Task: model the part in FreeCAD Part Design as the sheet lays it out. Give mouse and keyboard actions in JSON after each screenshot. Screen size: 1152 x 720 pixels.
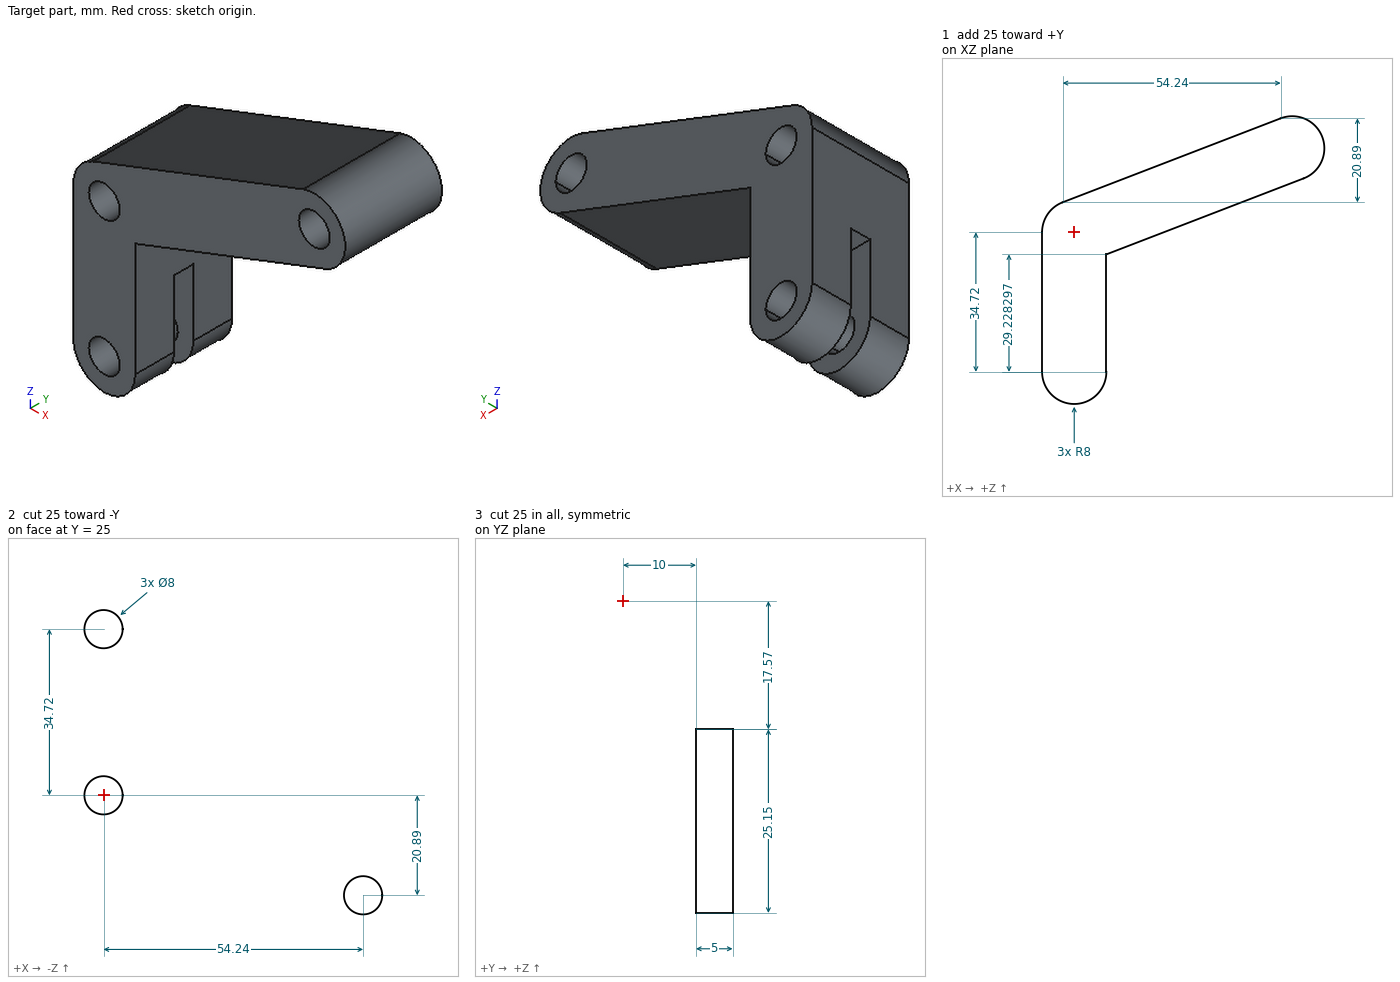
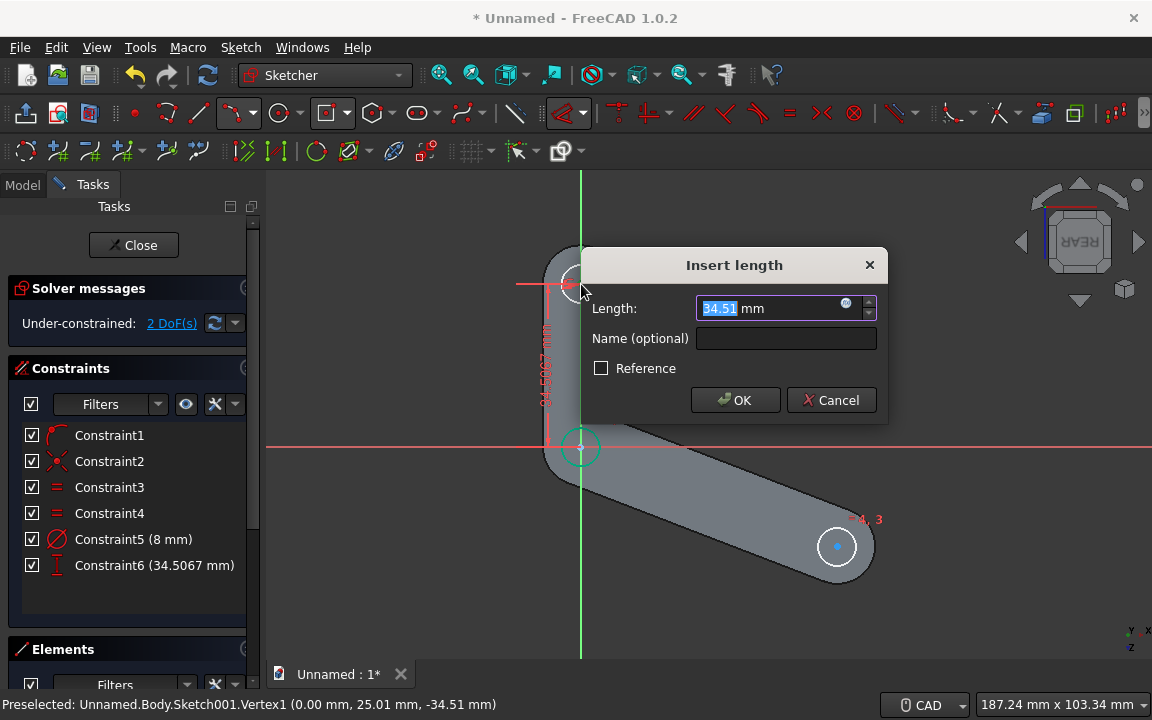
{"action": "type", "text": "34.72"}
{"action": "key", "text": "Return"}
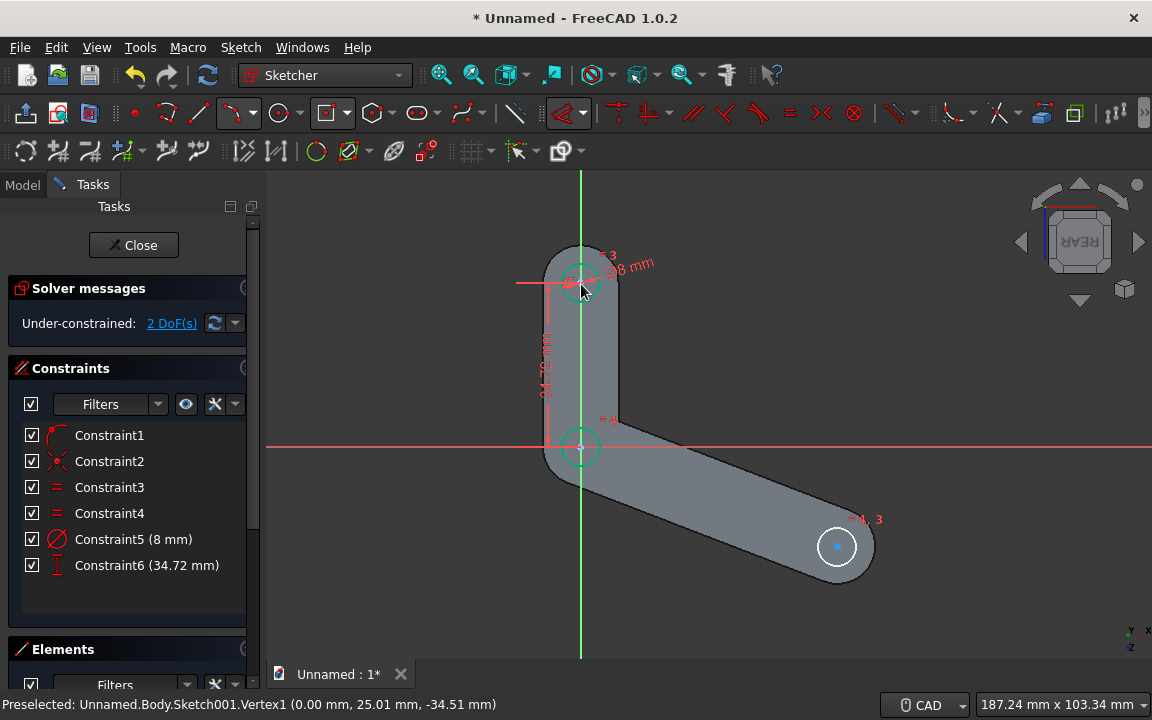
{"action": "left_click", "coordinate": [837, 547]}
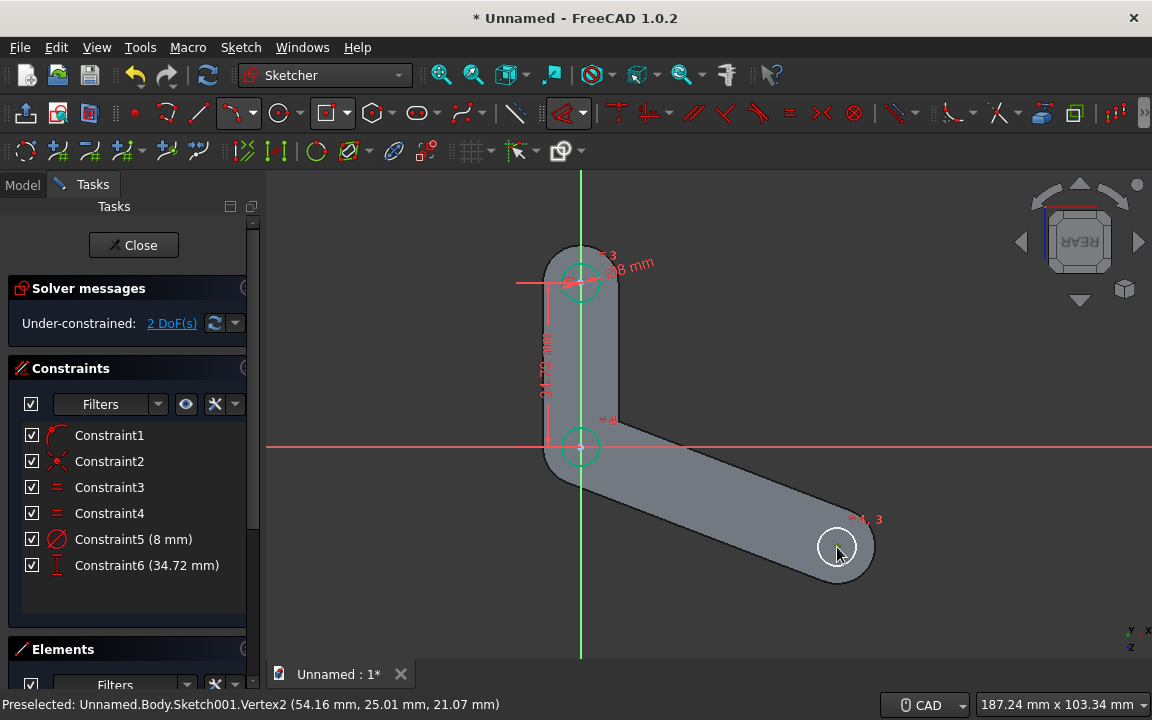
{"action": "key", "text": "l"}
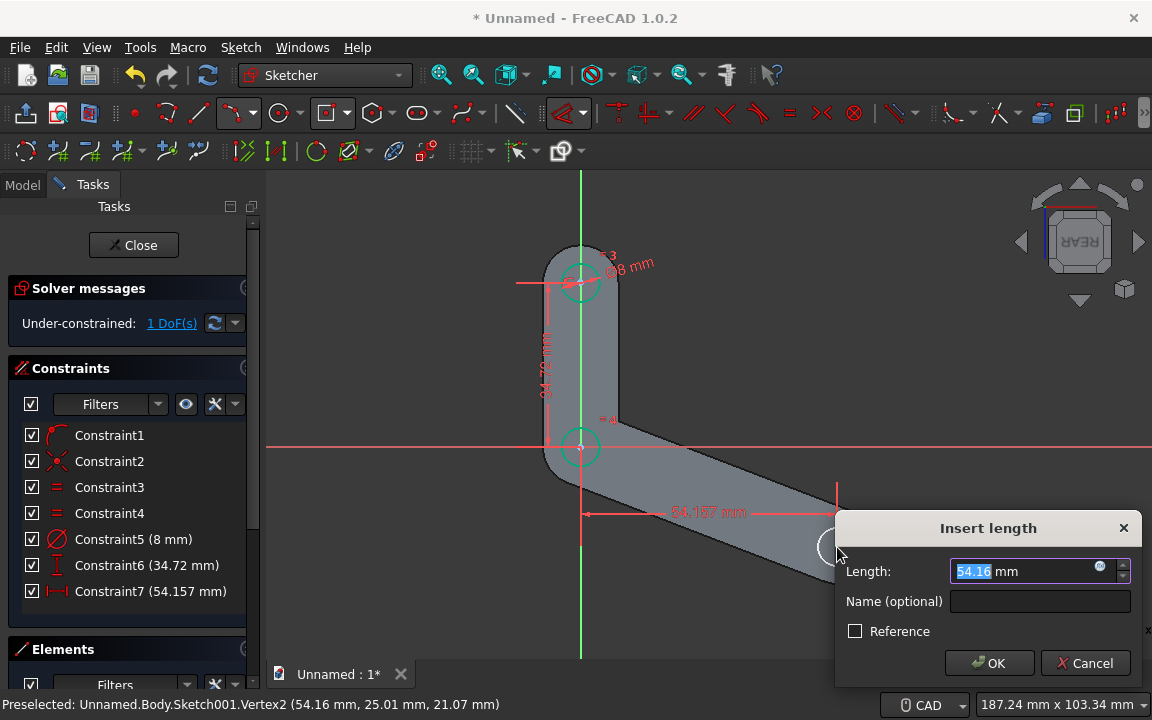
{"action": "type", "text": "54.24"}
{"action": "key", "text": "Return"}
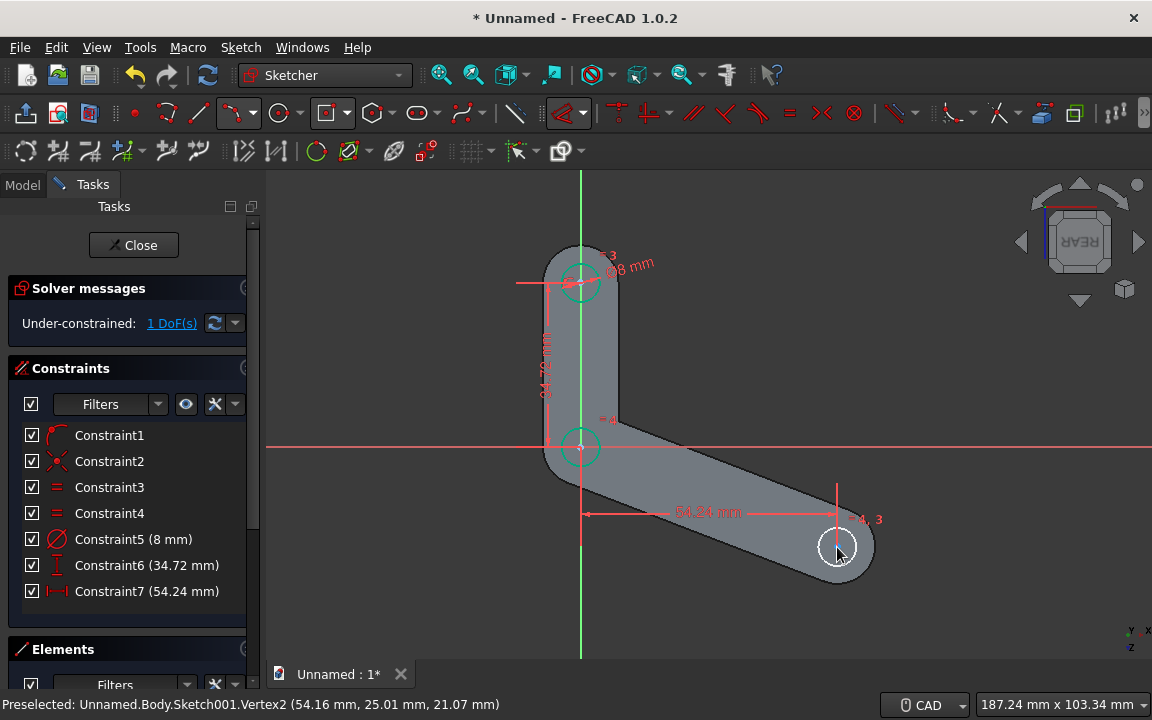
{"action": "left_click", "coordinate": [837, 547]}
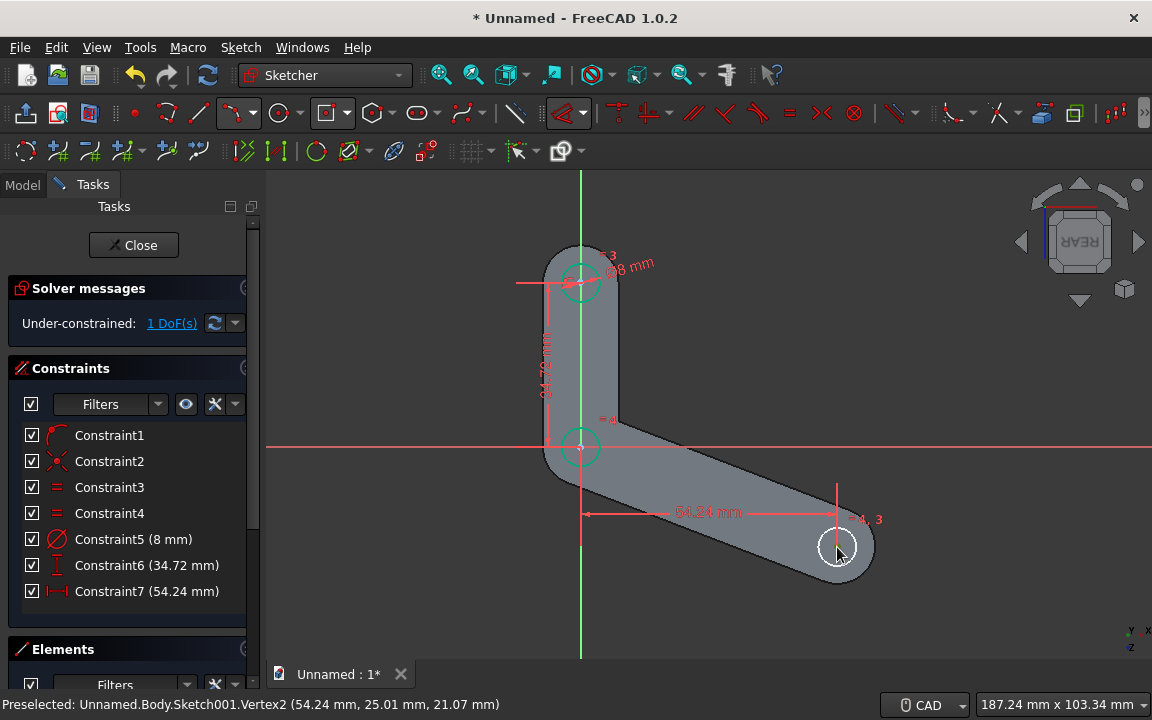
{"action": "left_click", "coordinate": [586, 114]}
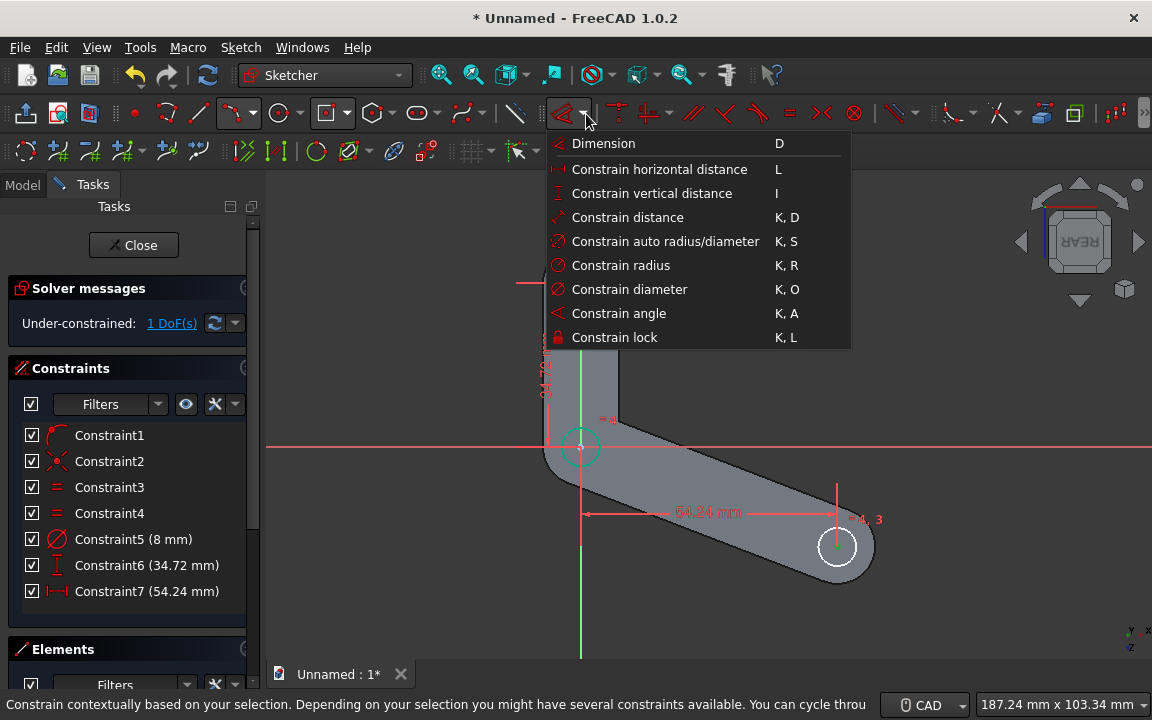
{"action": "left_click", "coordinate": [699, 193]}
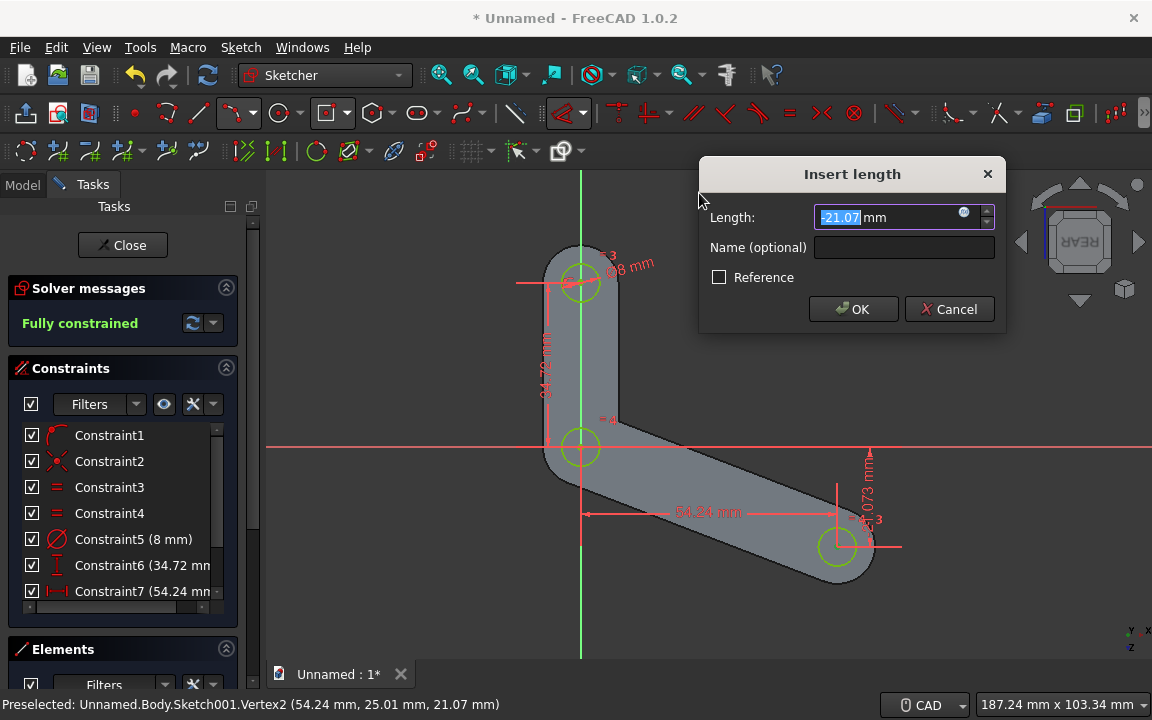
{"action": "type", "text": "-20.89"}
{"action": "key", "text": "Return"}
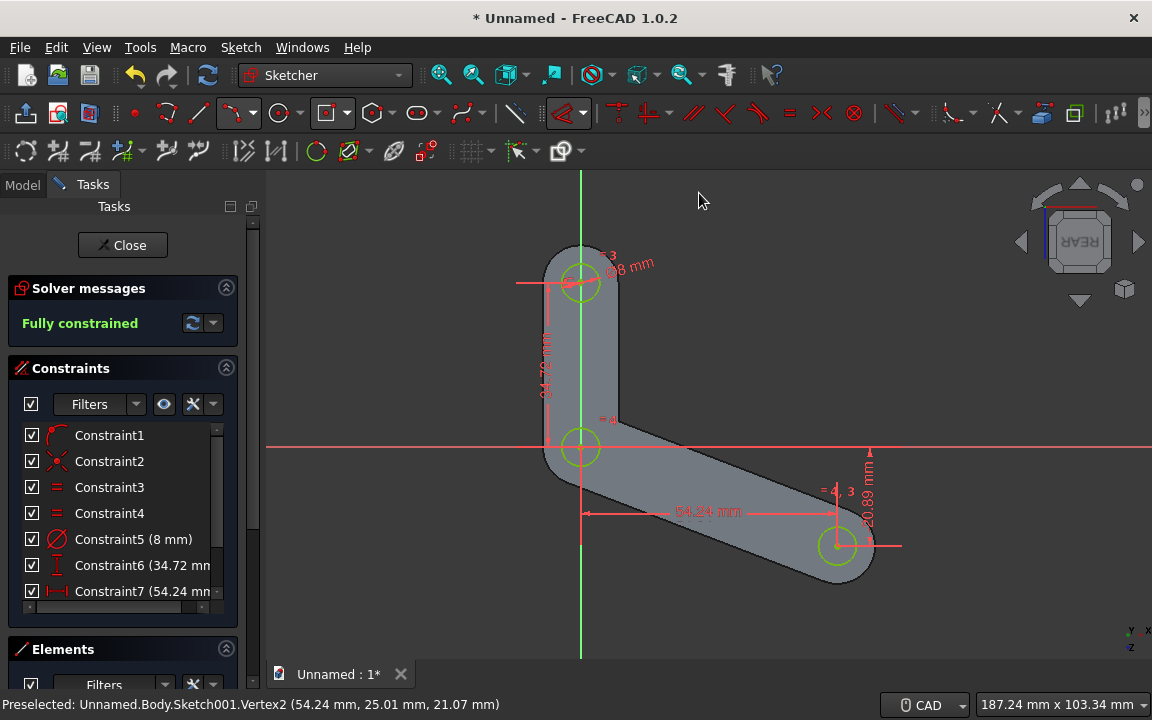
{"action": "left_click", "coordinate": [123, 245]}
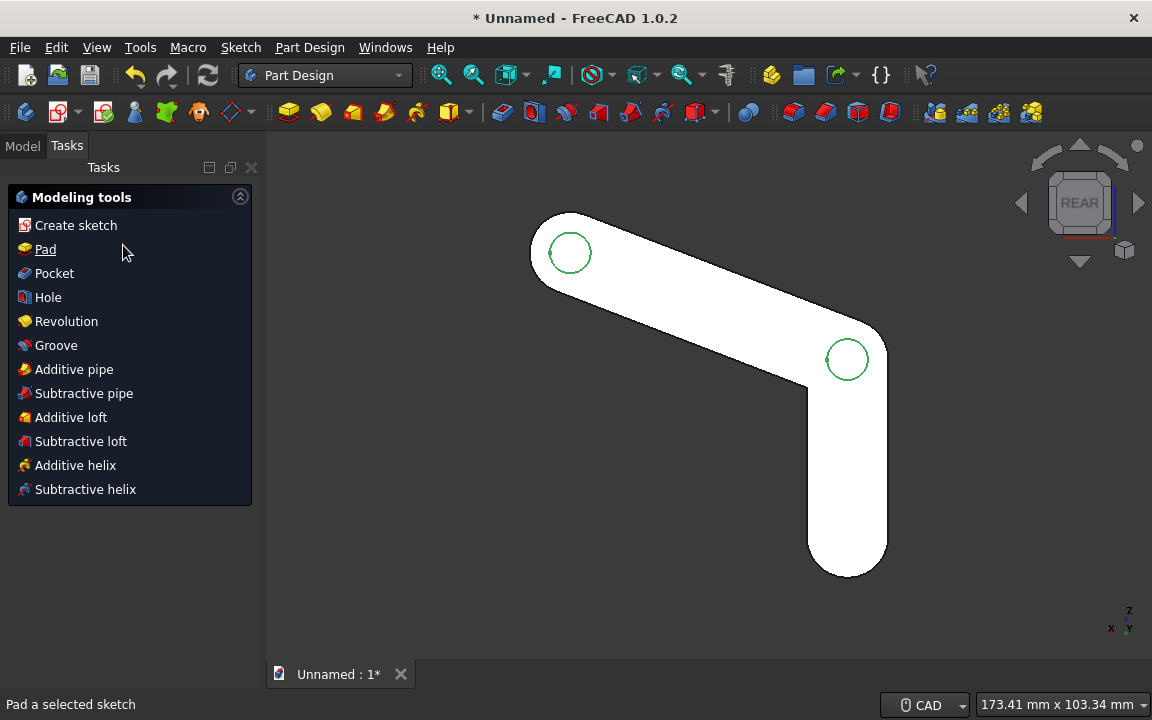
{"action": "left_click", "coordinate": [504, 112]}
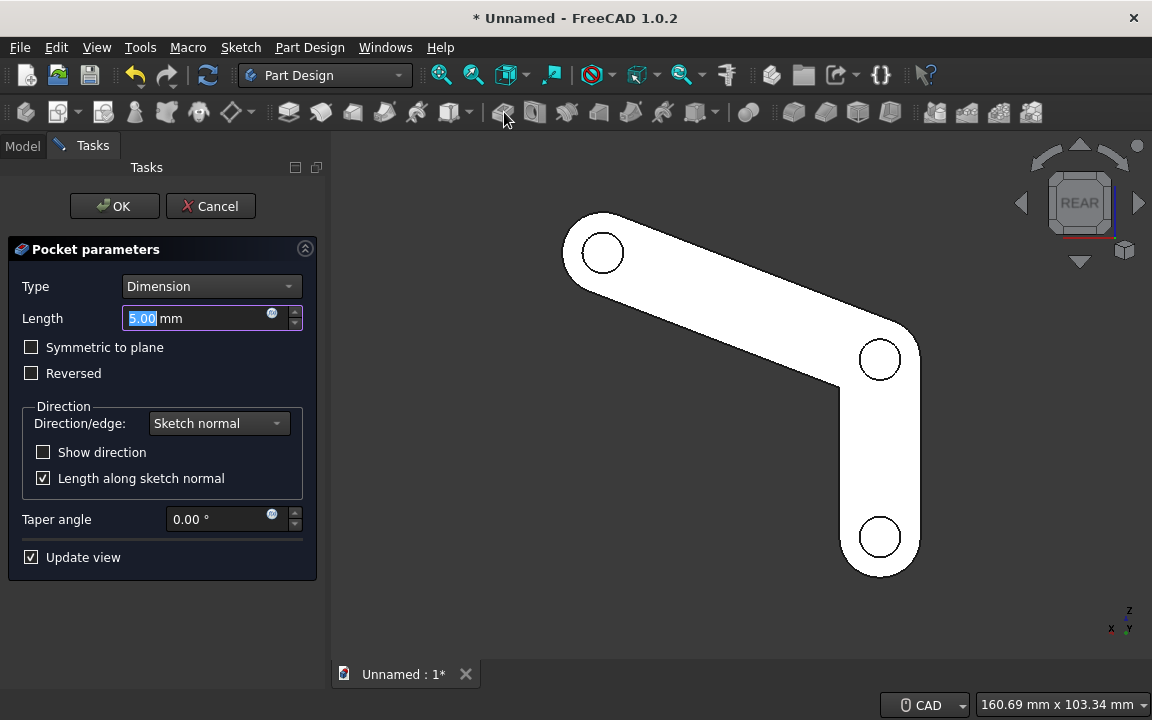
{"action": "type", "text": "25"}
{"action": "key", "text": "Tab"}